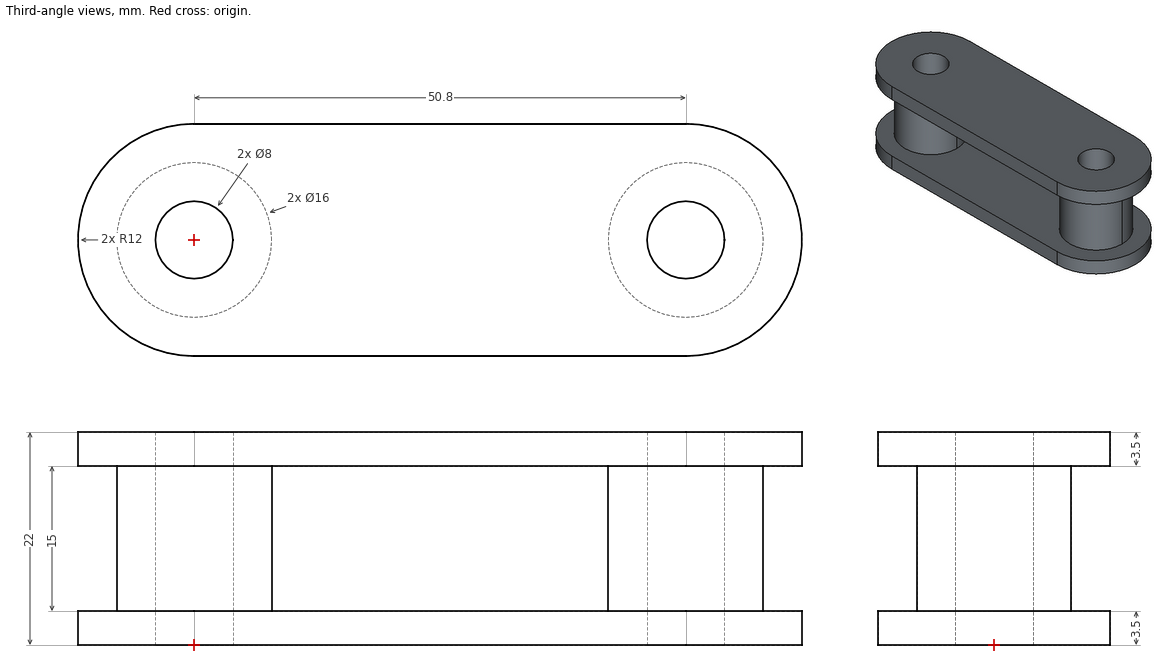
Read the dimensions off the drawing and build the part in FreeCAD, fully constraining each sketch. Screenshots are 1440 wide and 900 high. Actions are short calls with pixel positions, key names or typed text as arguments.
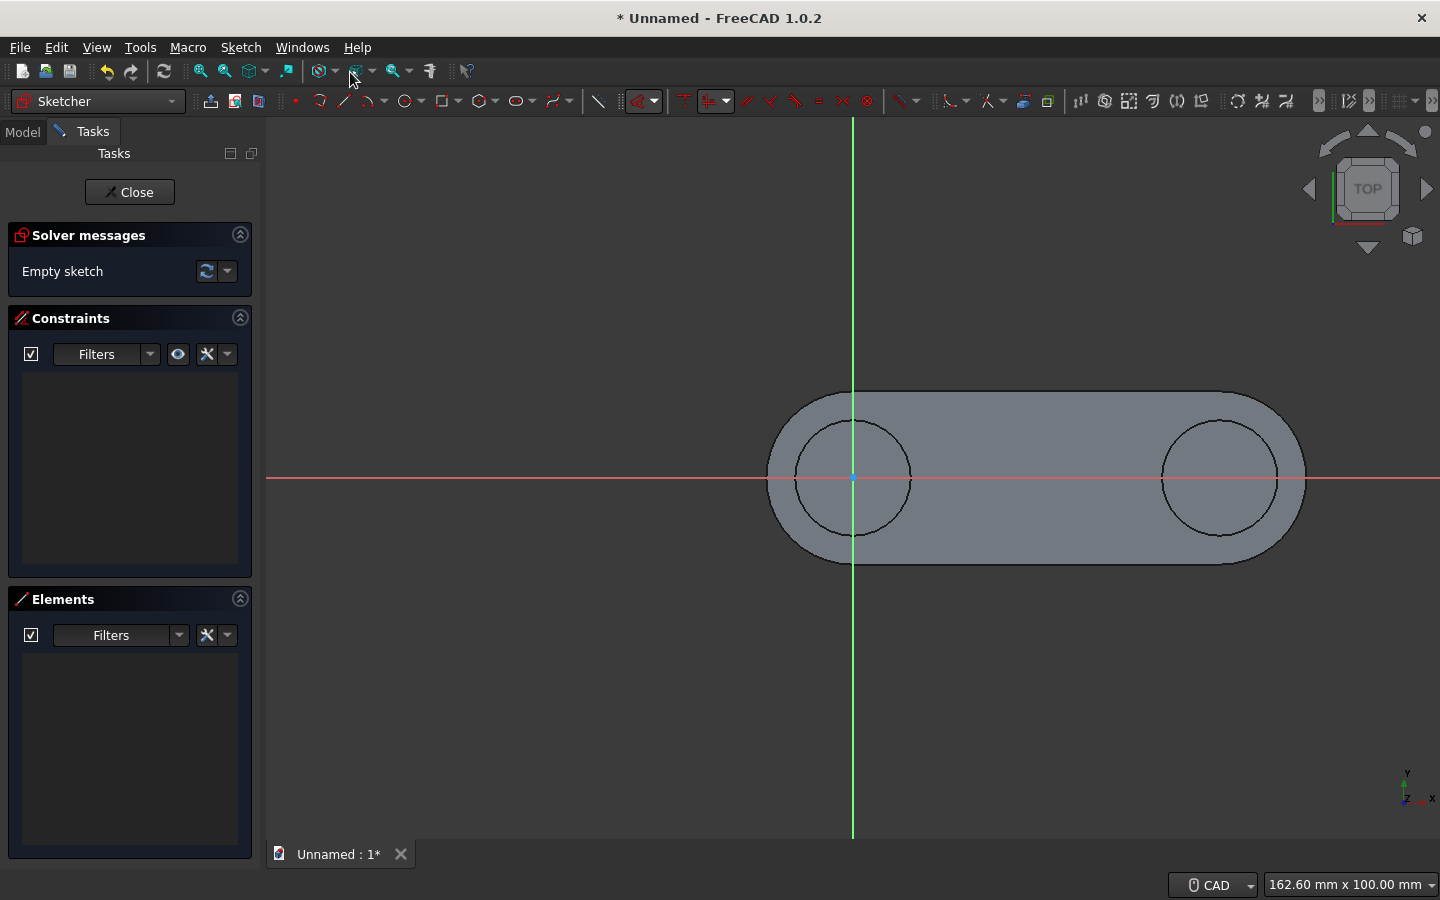
scroll(294, 478, down, 1)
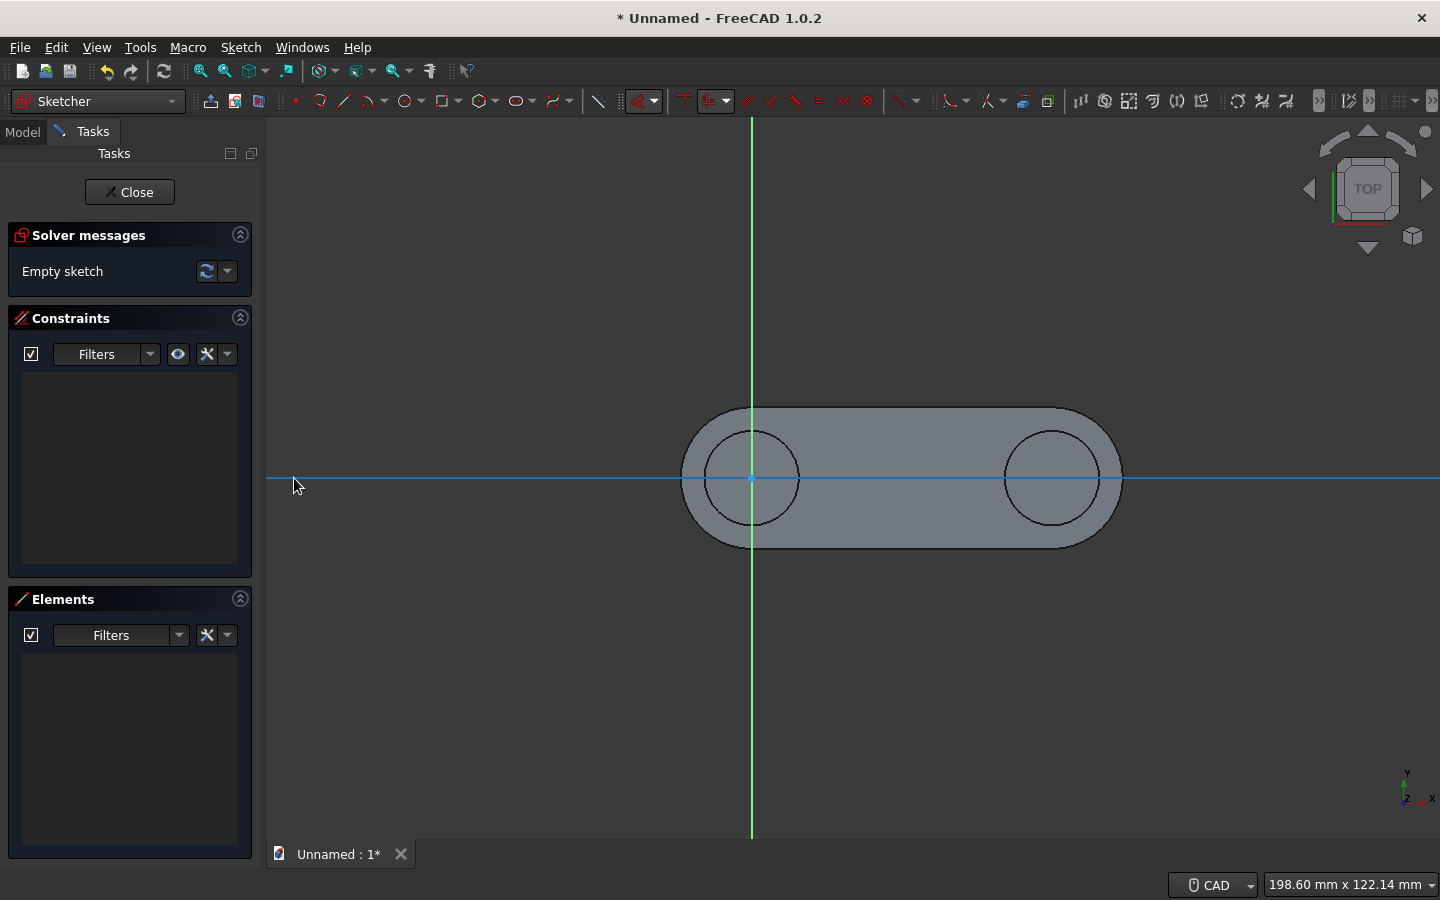
scroll(1140, 478, up, 2)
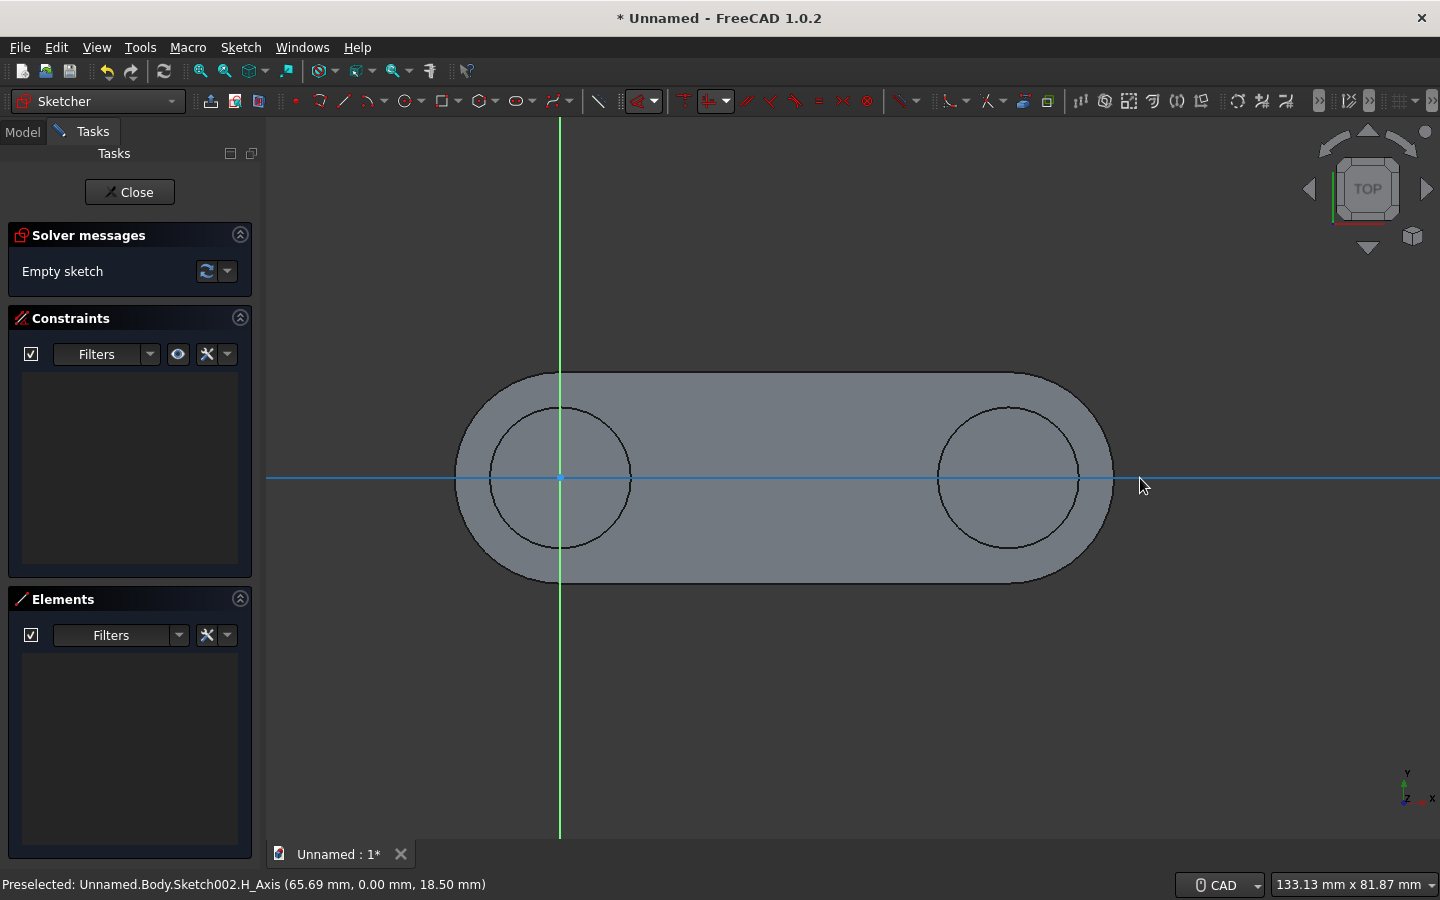
click(516, 102)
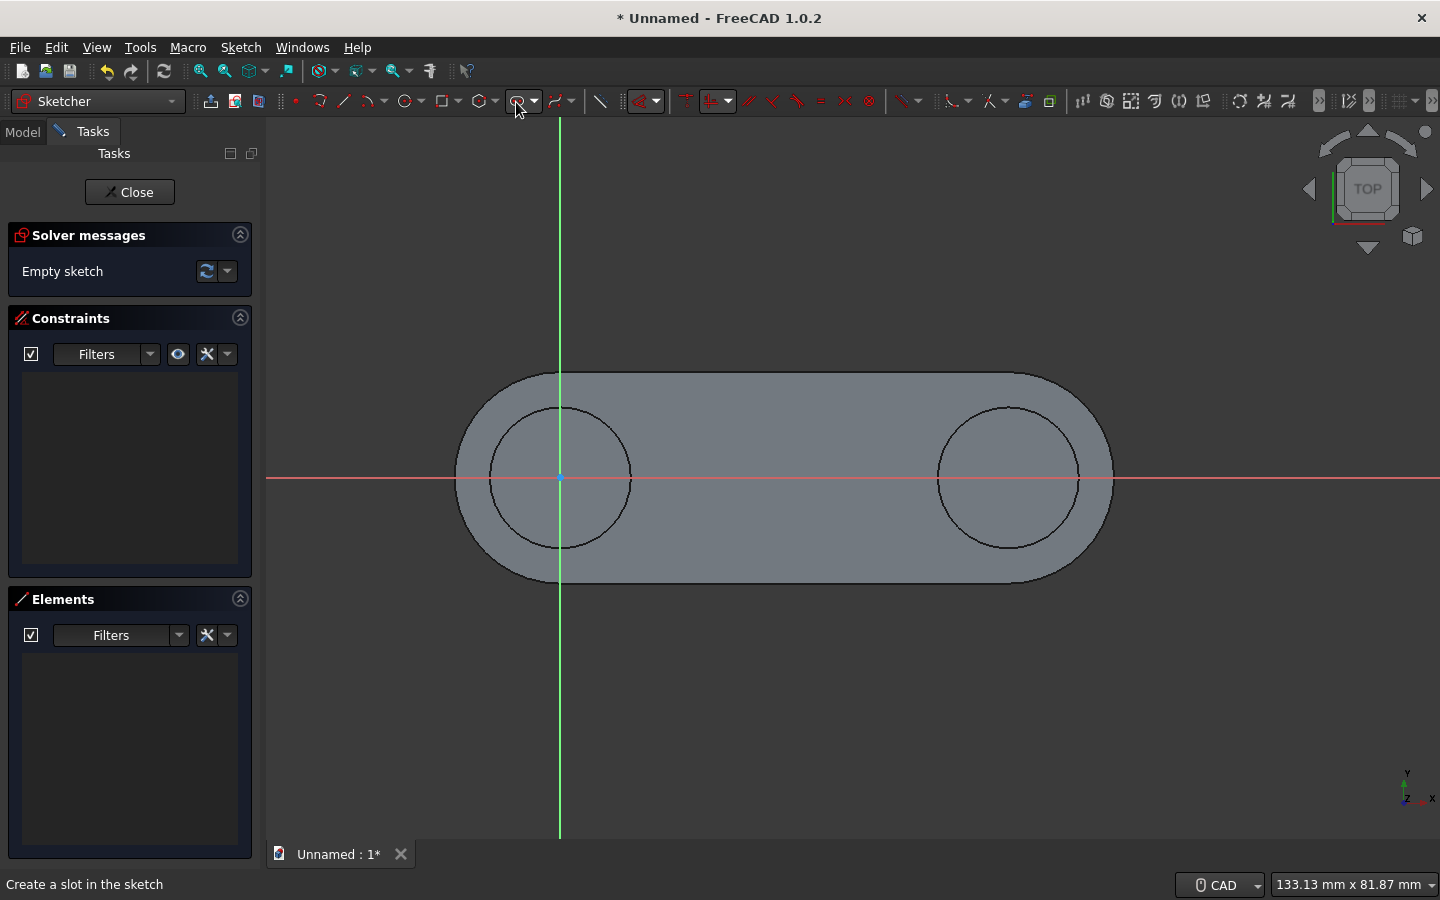
click(560, 478)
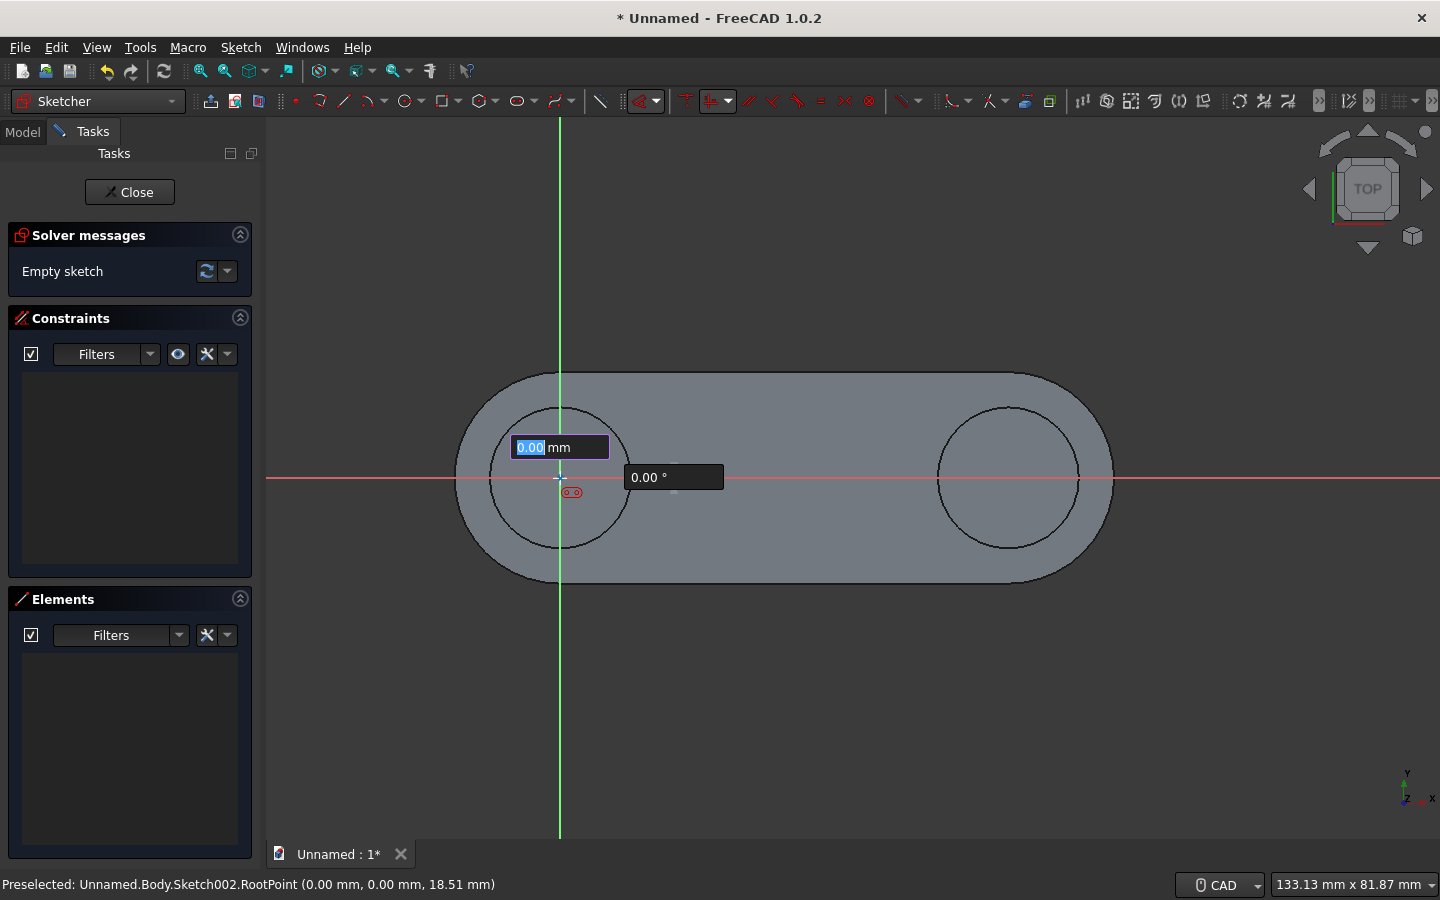
click(1008, 469)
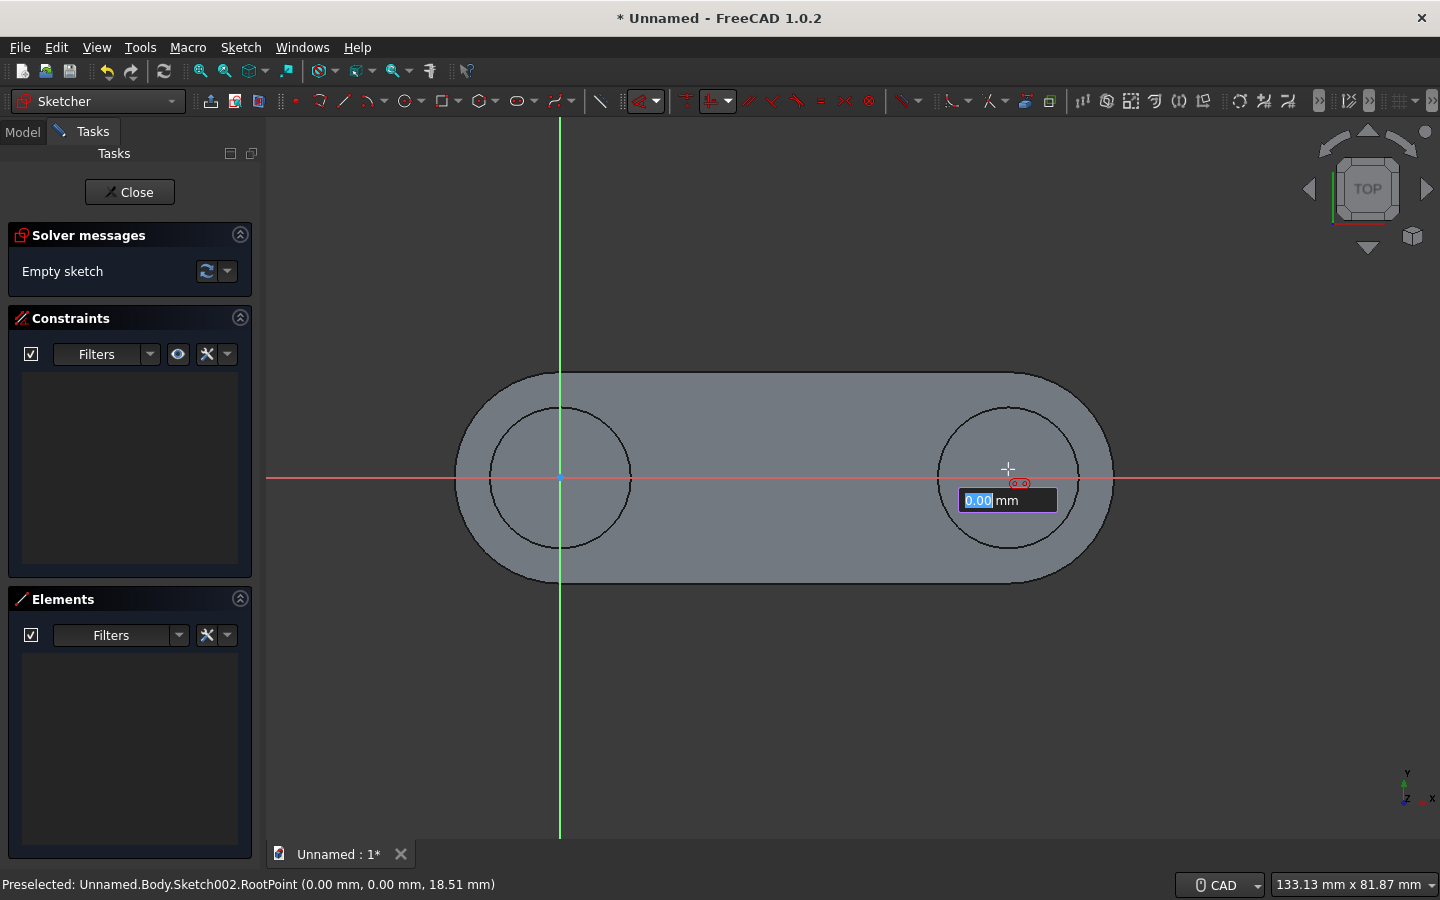
click(784, 372)
key(Escape)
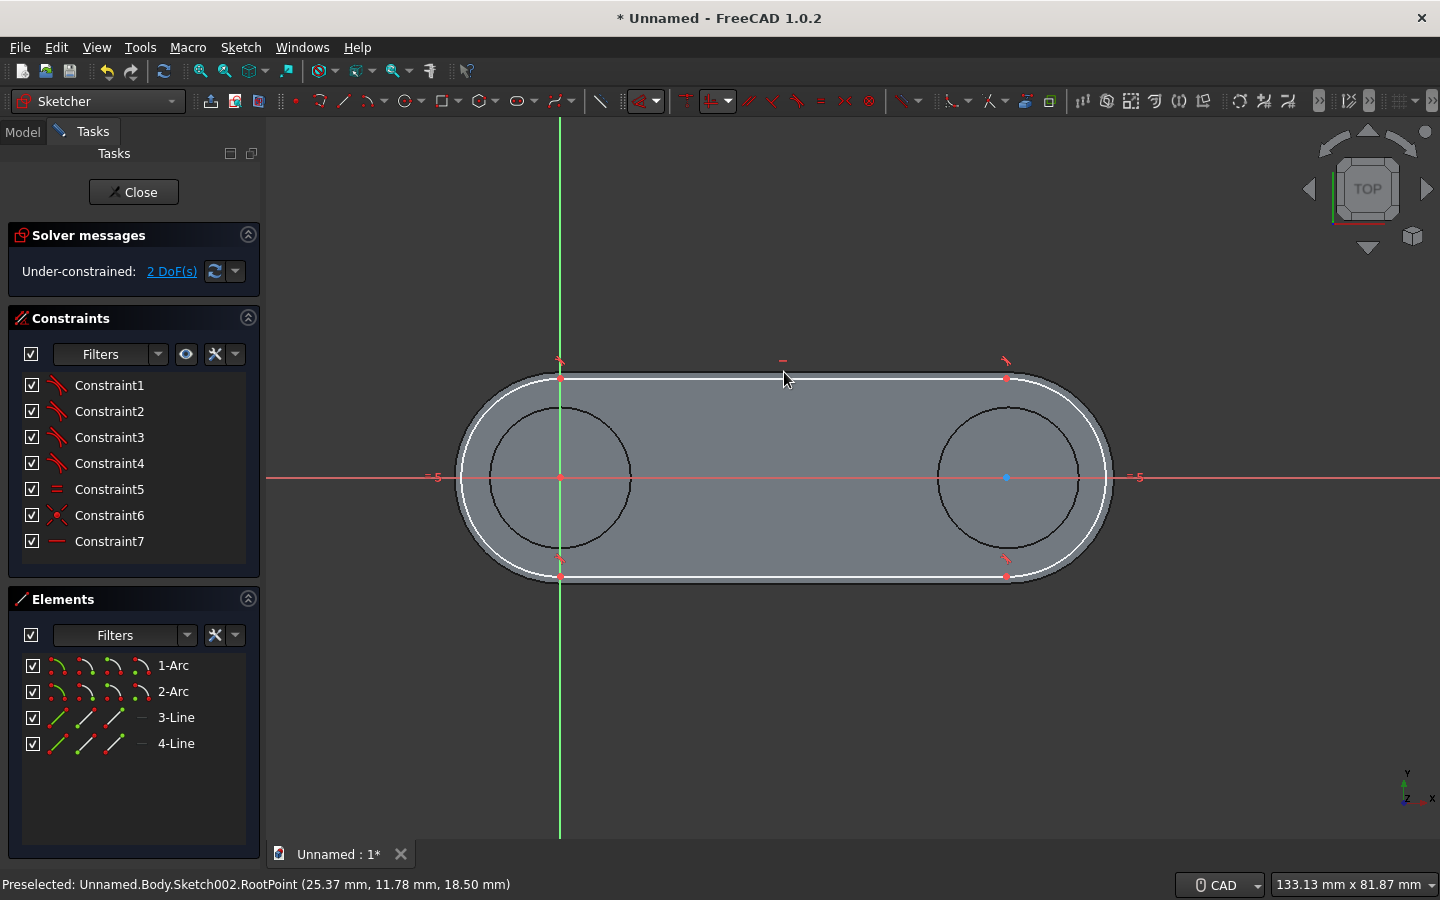
click(480, 420)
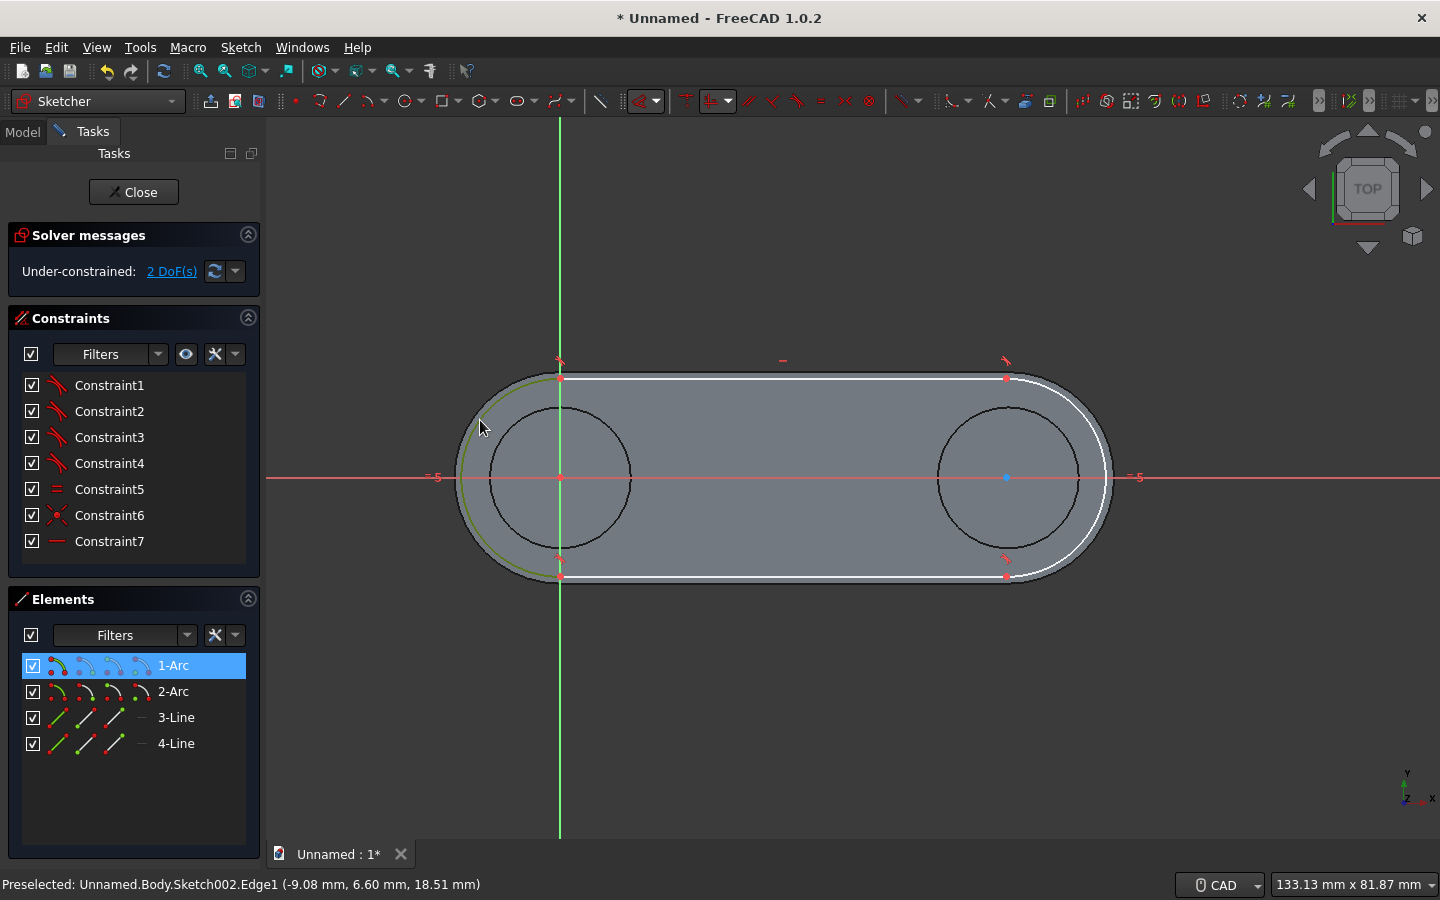
key(k)
key(r)